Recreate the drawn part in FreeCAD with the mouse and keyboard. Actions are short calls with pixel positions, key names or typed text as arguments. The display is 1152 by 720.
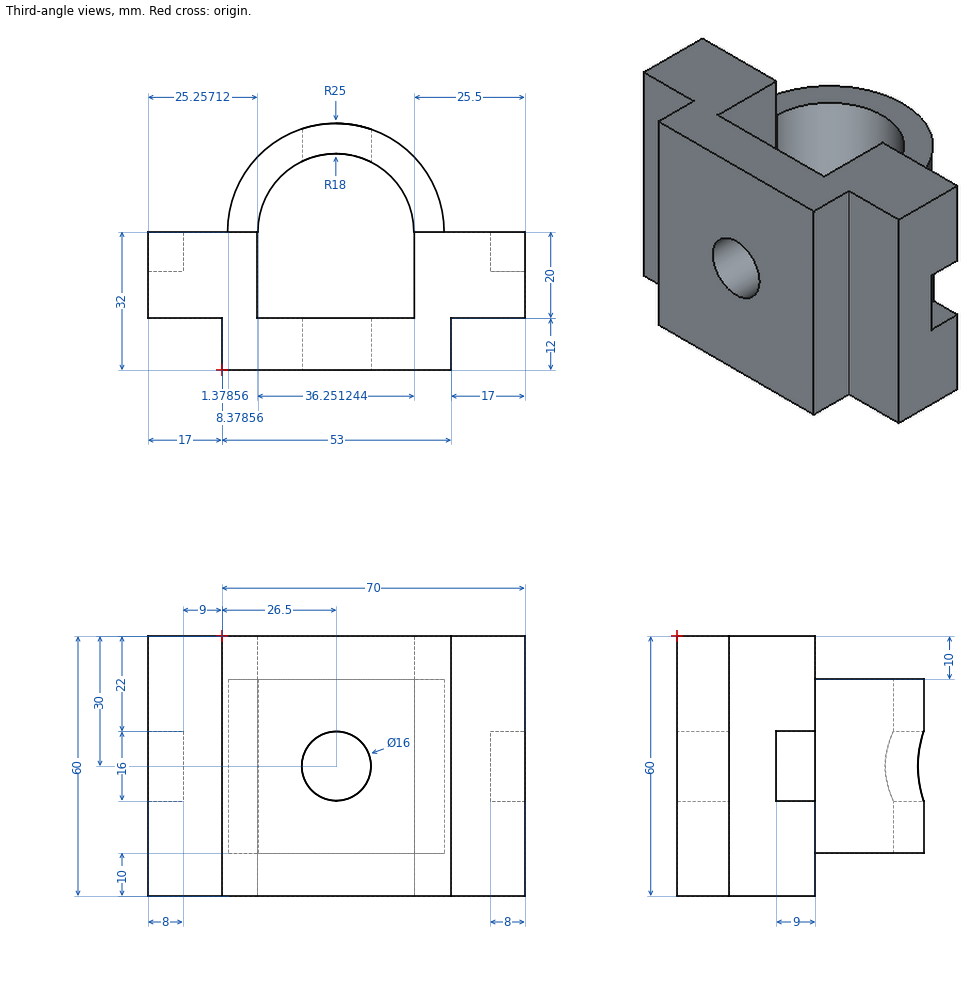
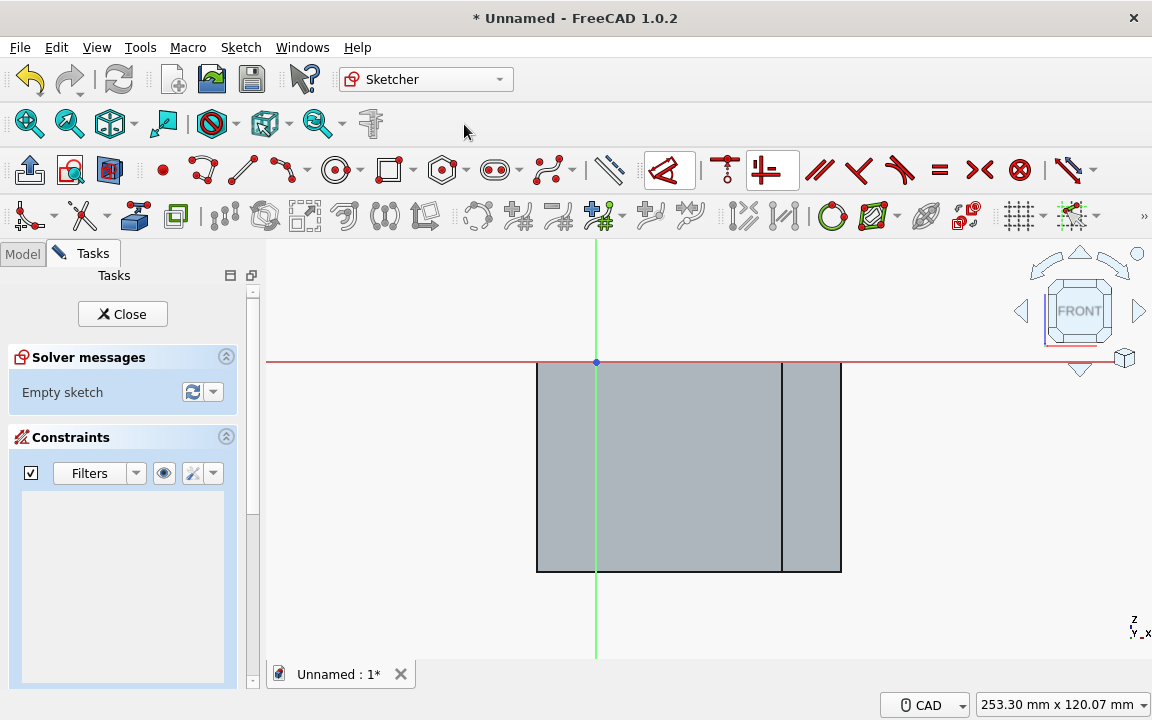
scroll(676, 404, up, 3)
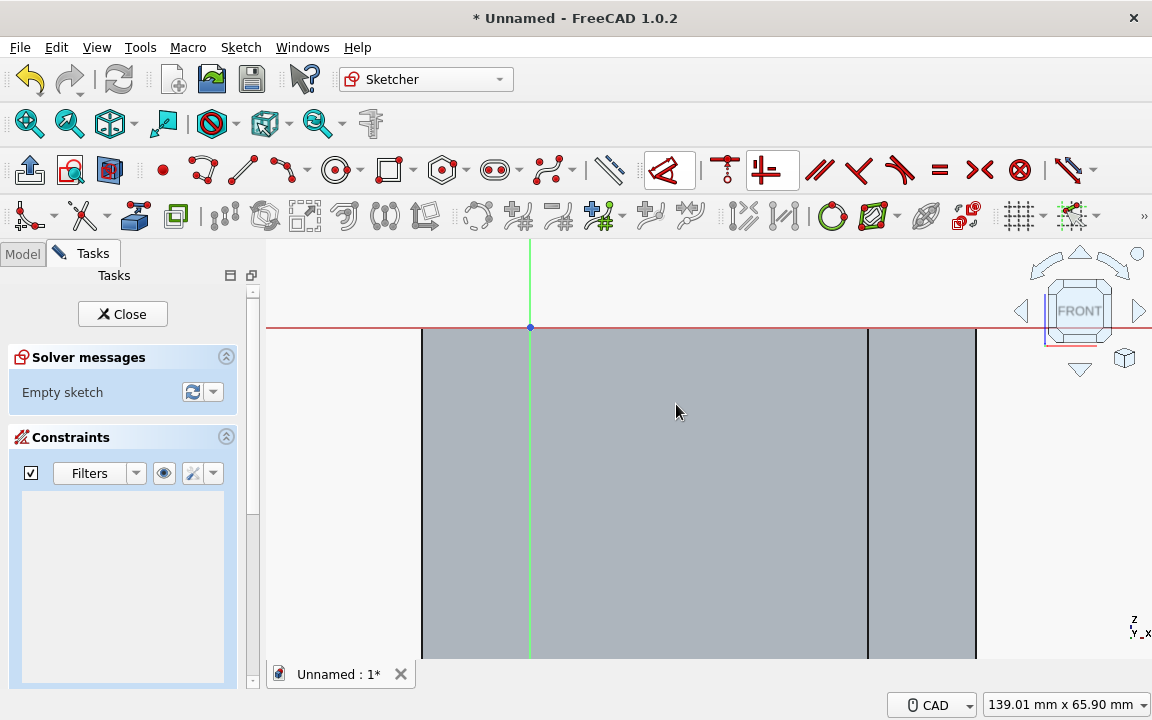
key(g)
key(c)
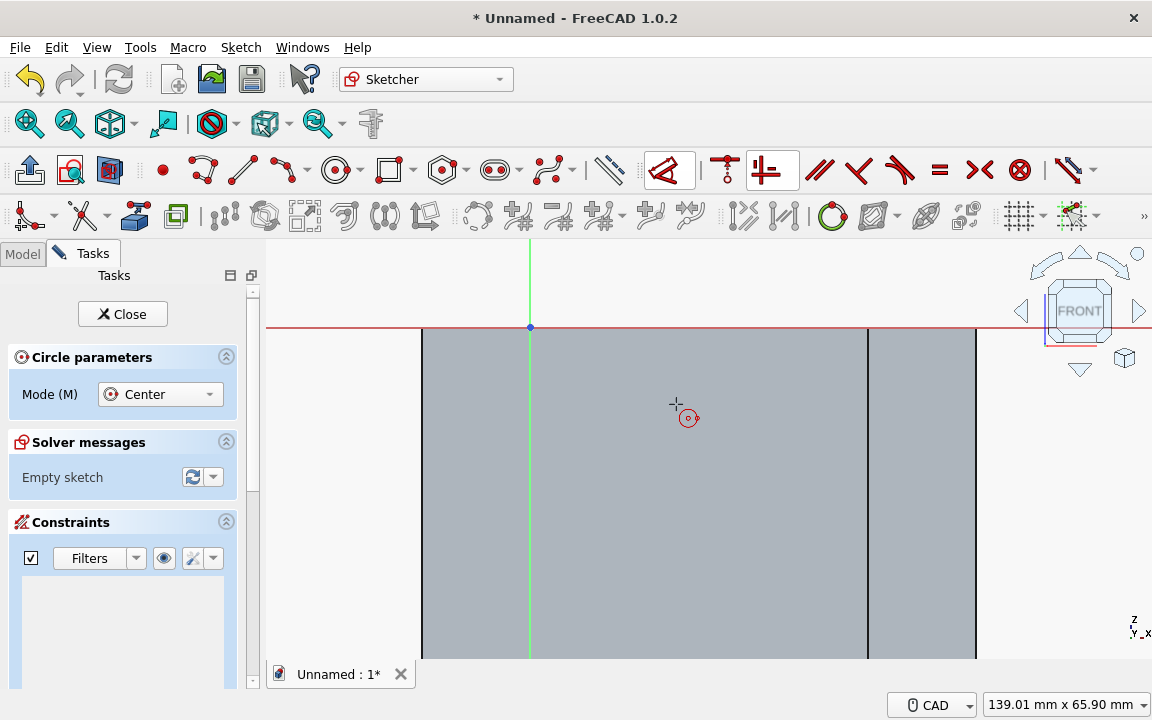
click(699, 519)
click(735, 483)
key(Escape)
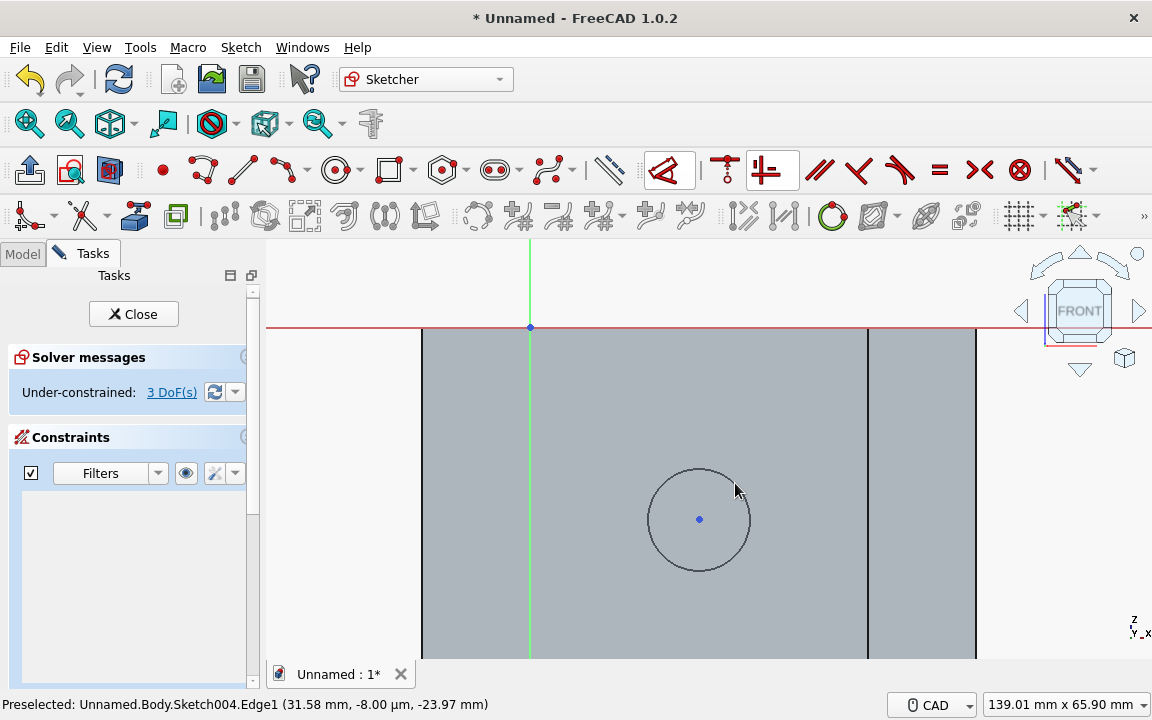
click(735, 484)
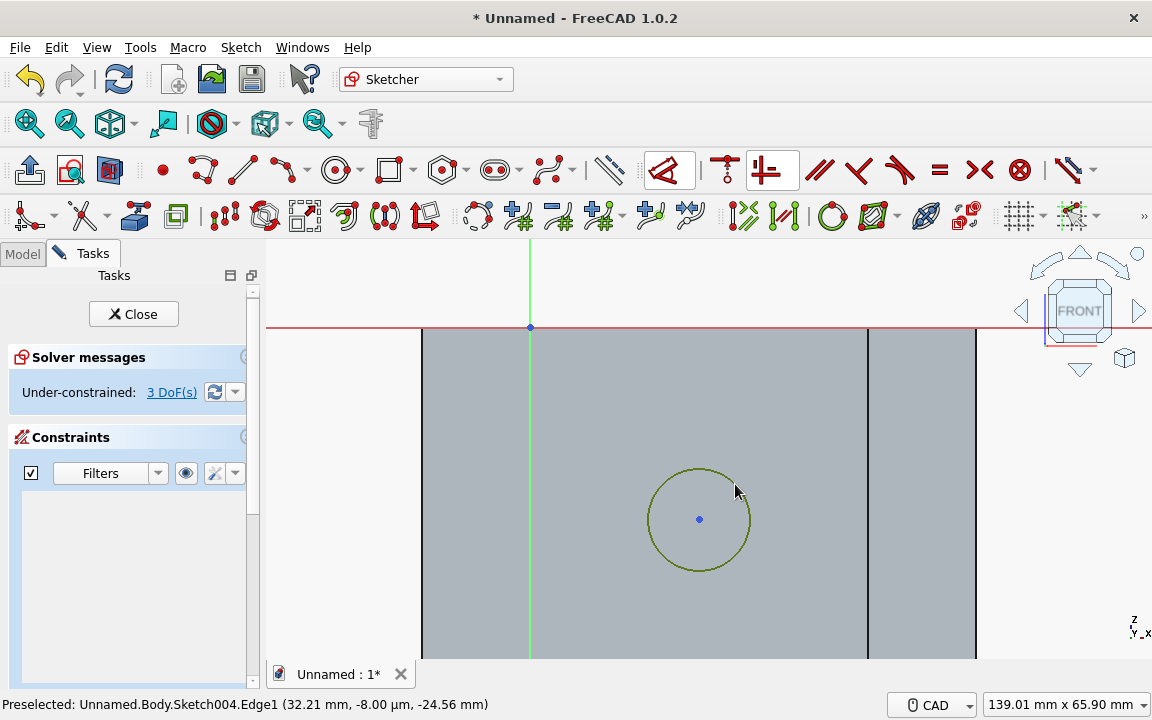
key(k)
key(o)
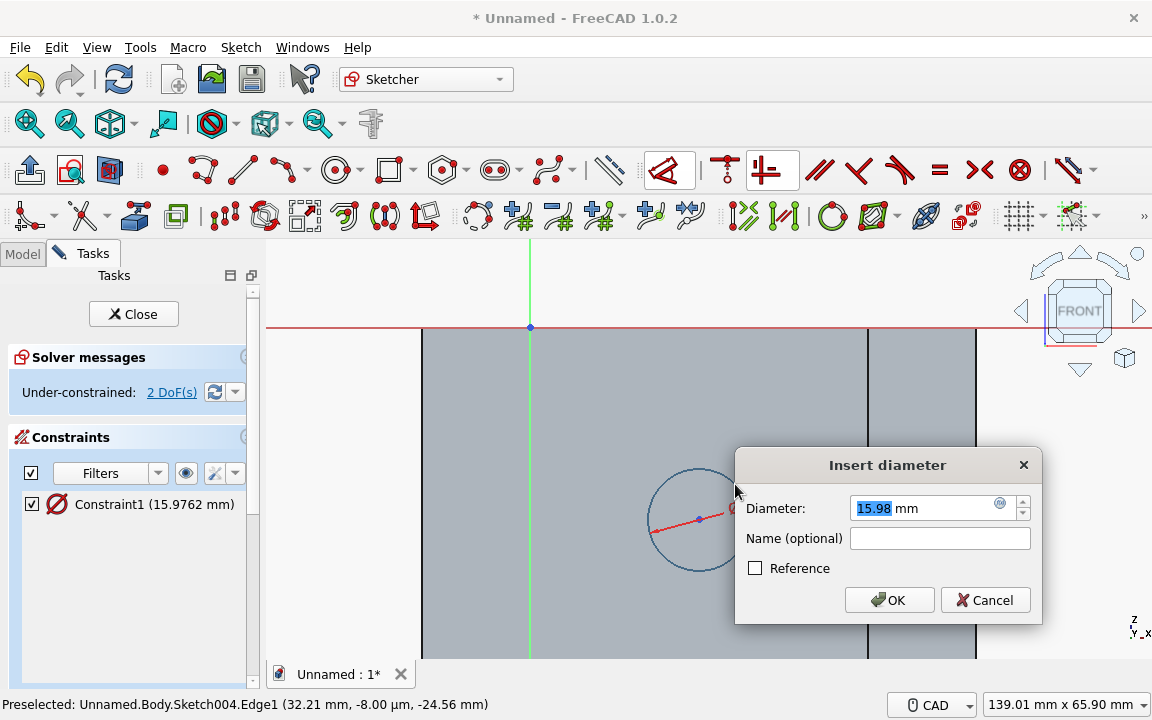
text(16)
key(Return)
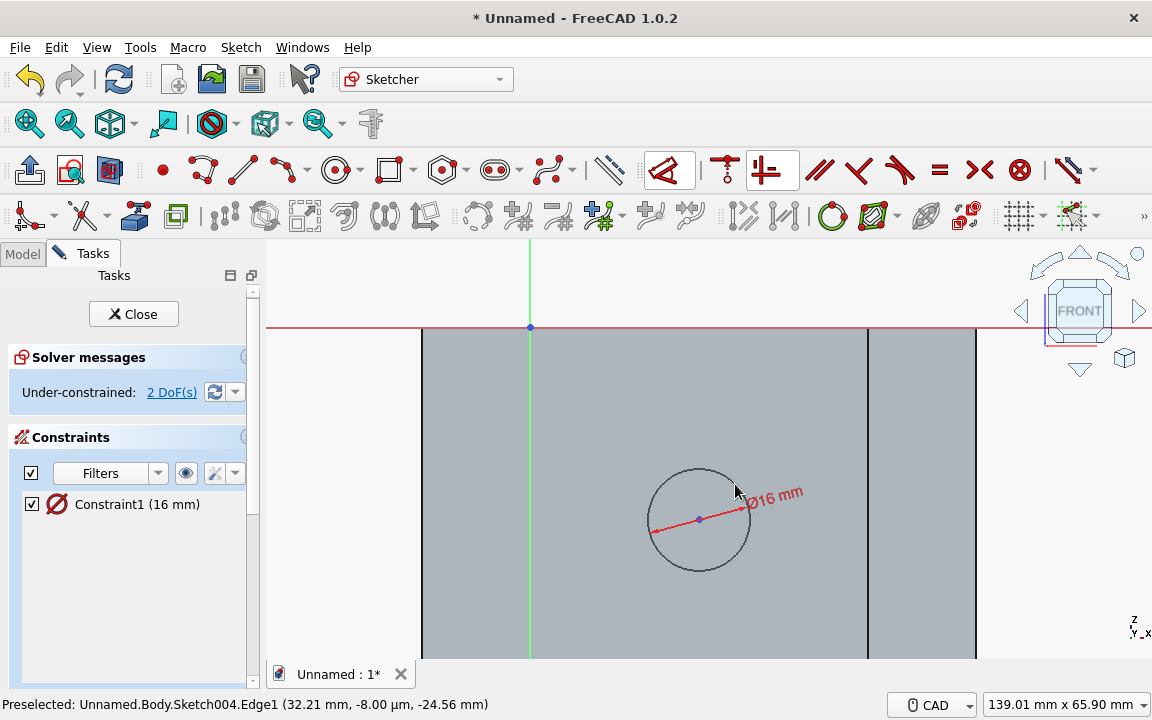
click(699, 520)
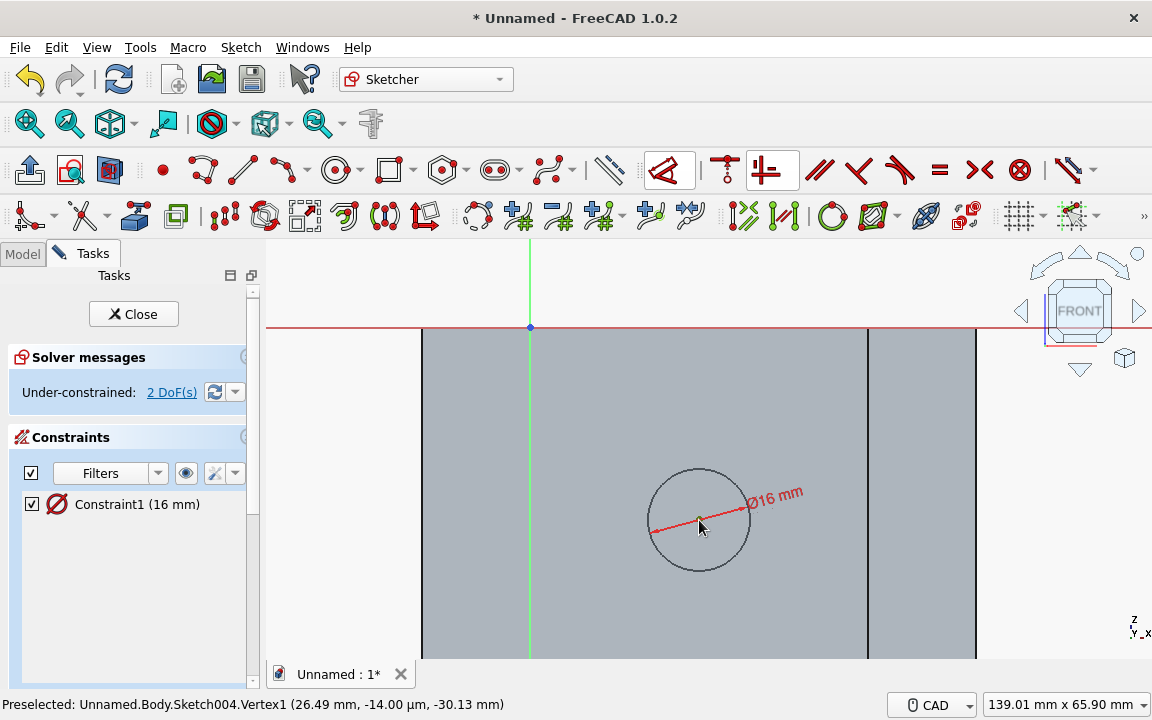
key(i)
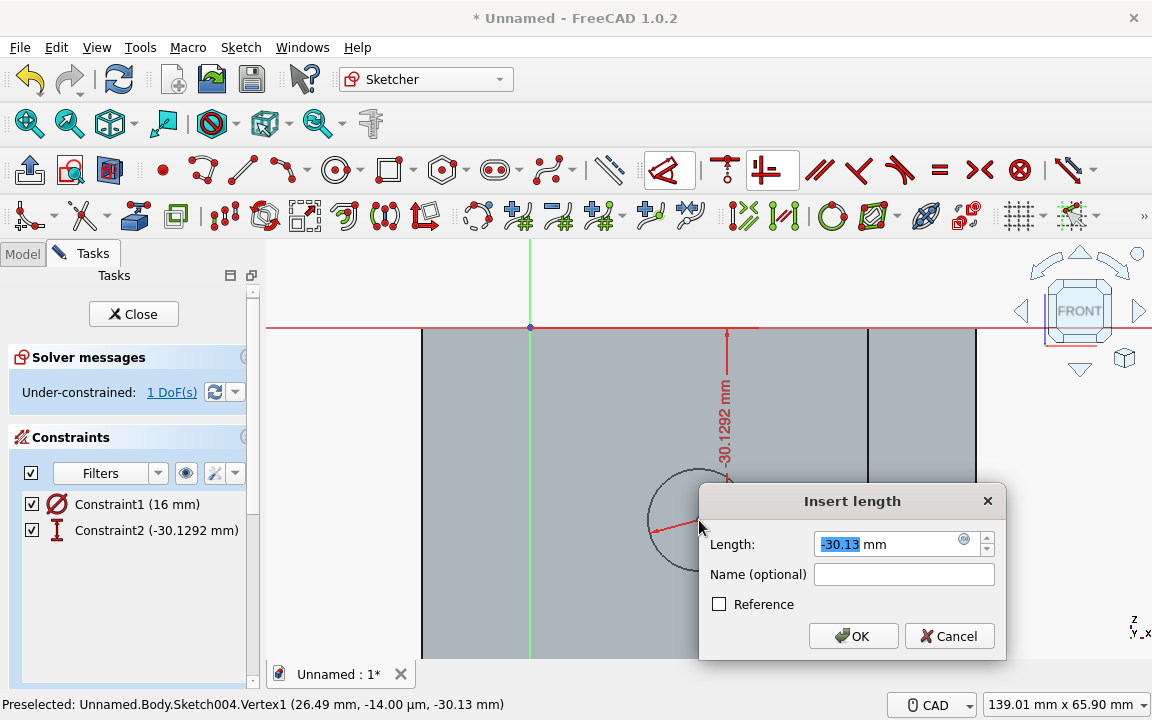
text(-30)
key(Return)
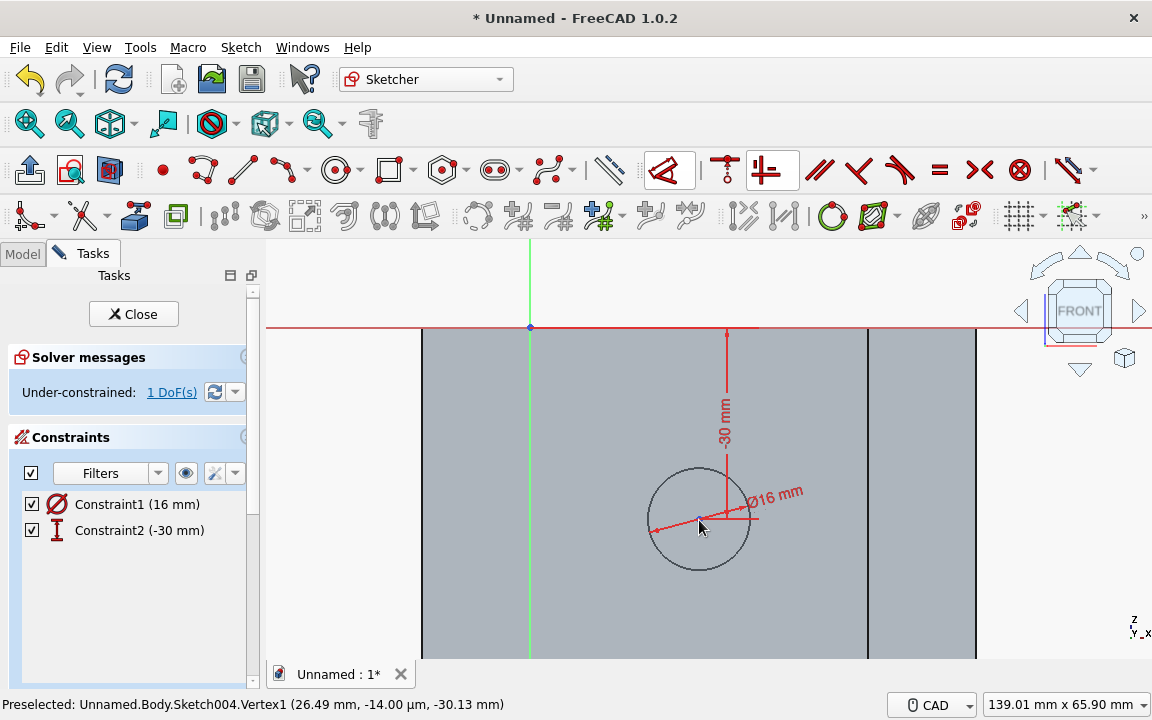
click(699, 519)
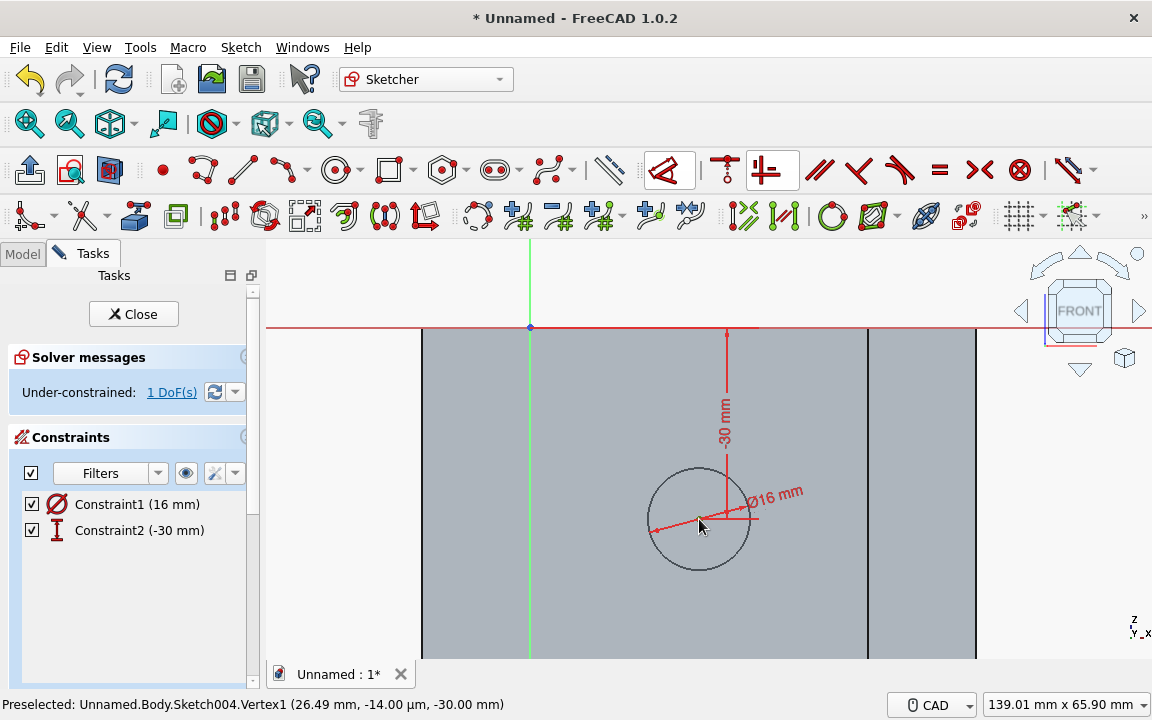
key(l)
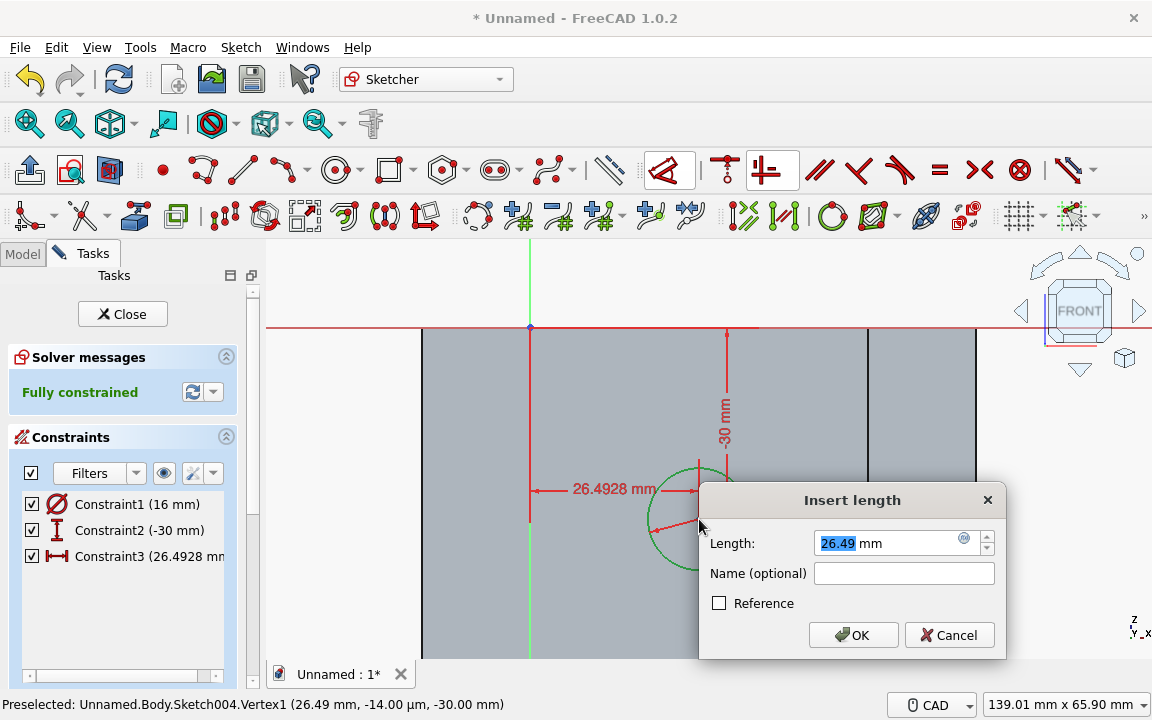
text(26.5)
key(Return)